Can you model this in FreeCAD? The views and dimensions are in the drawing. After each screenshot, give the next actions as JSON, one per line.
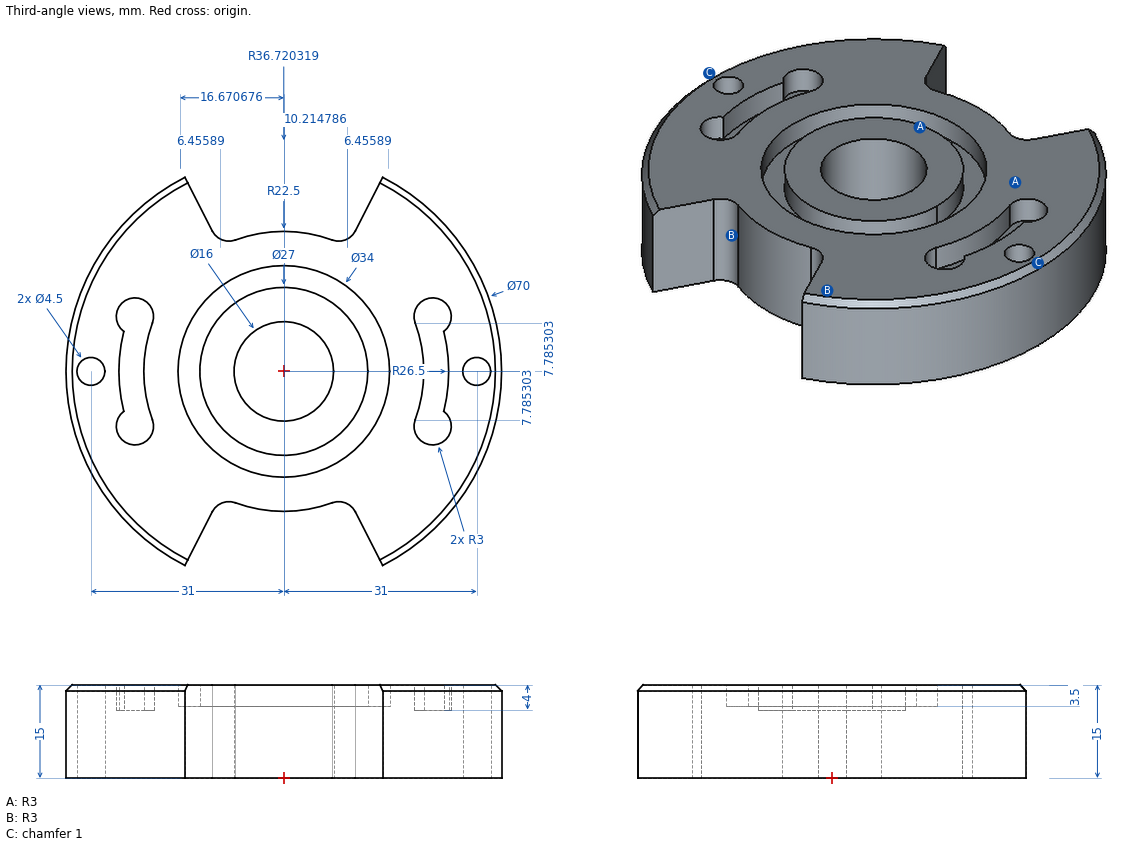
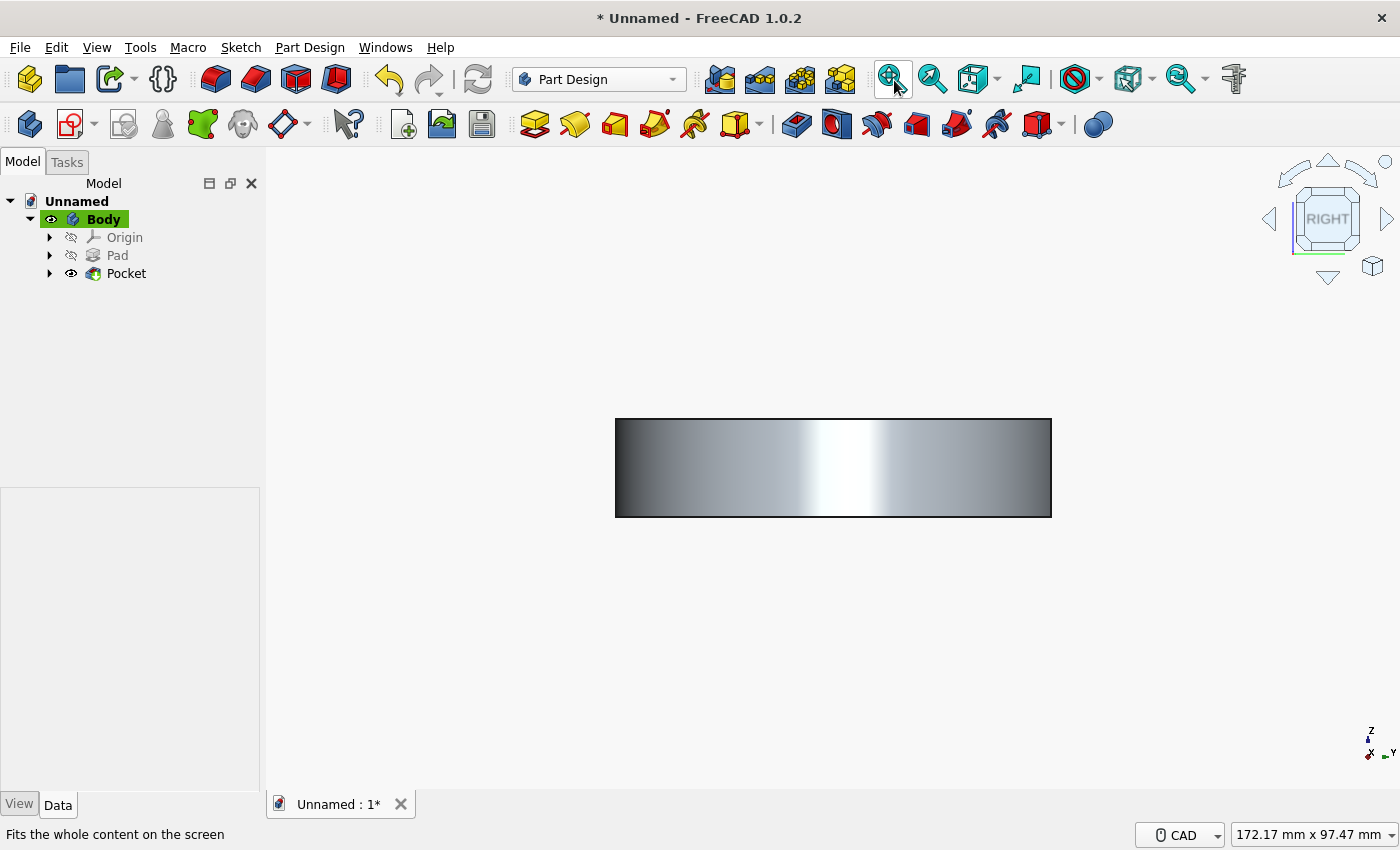
{"action": "key", "text": "5"}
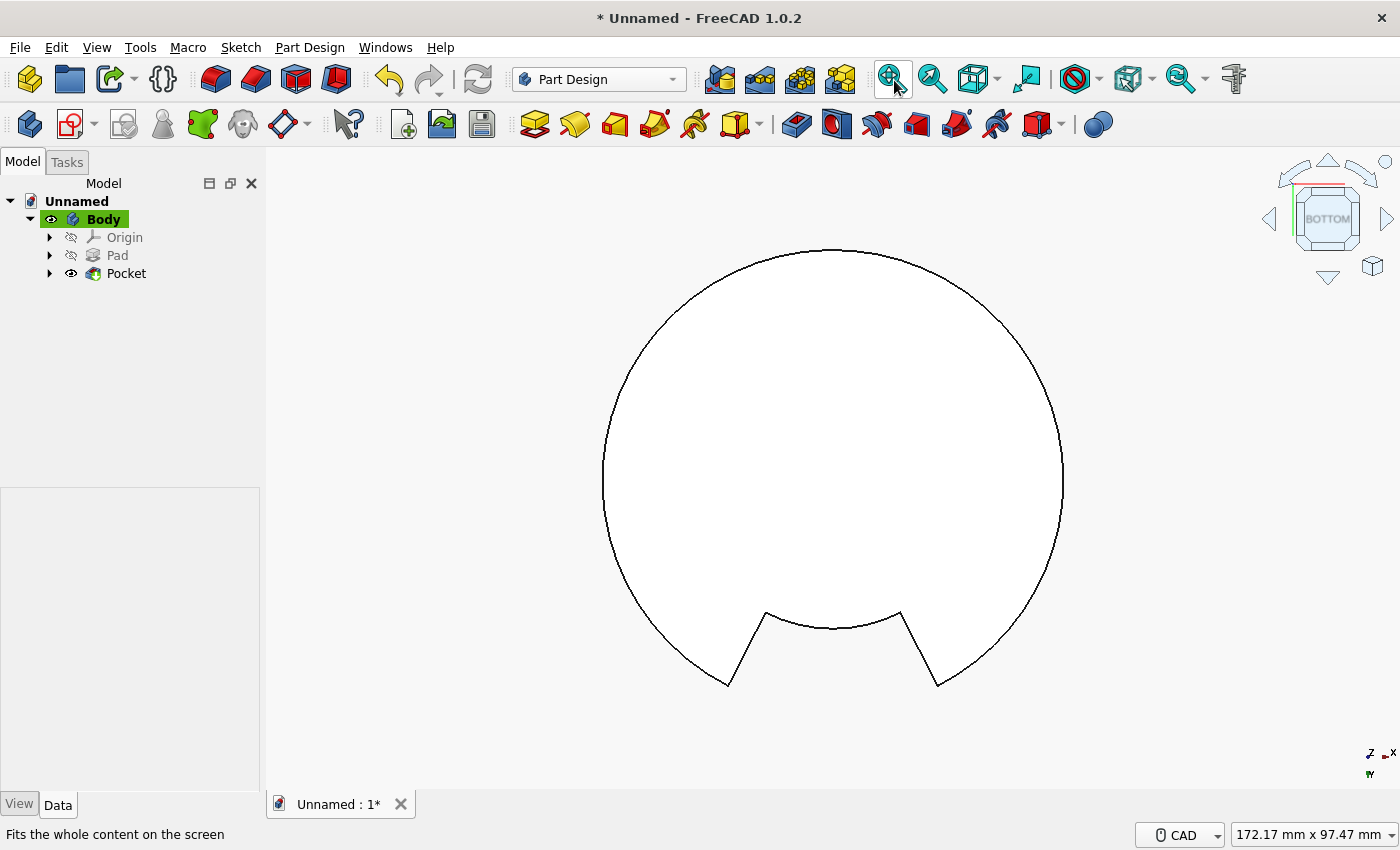
{"action": "key", "text": "4"}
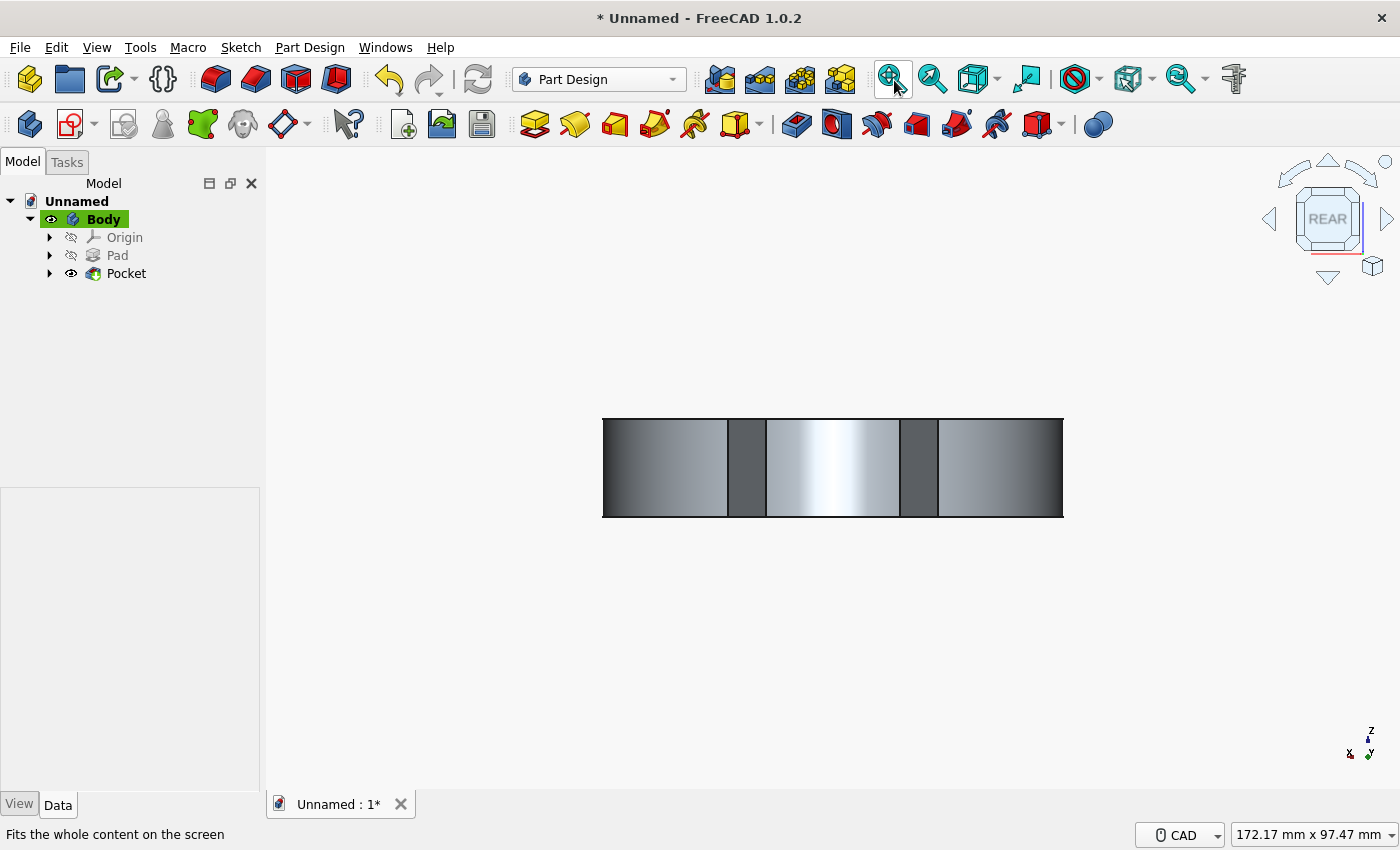
{"action": "key", "text": "v f"}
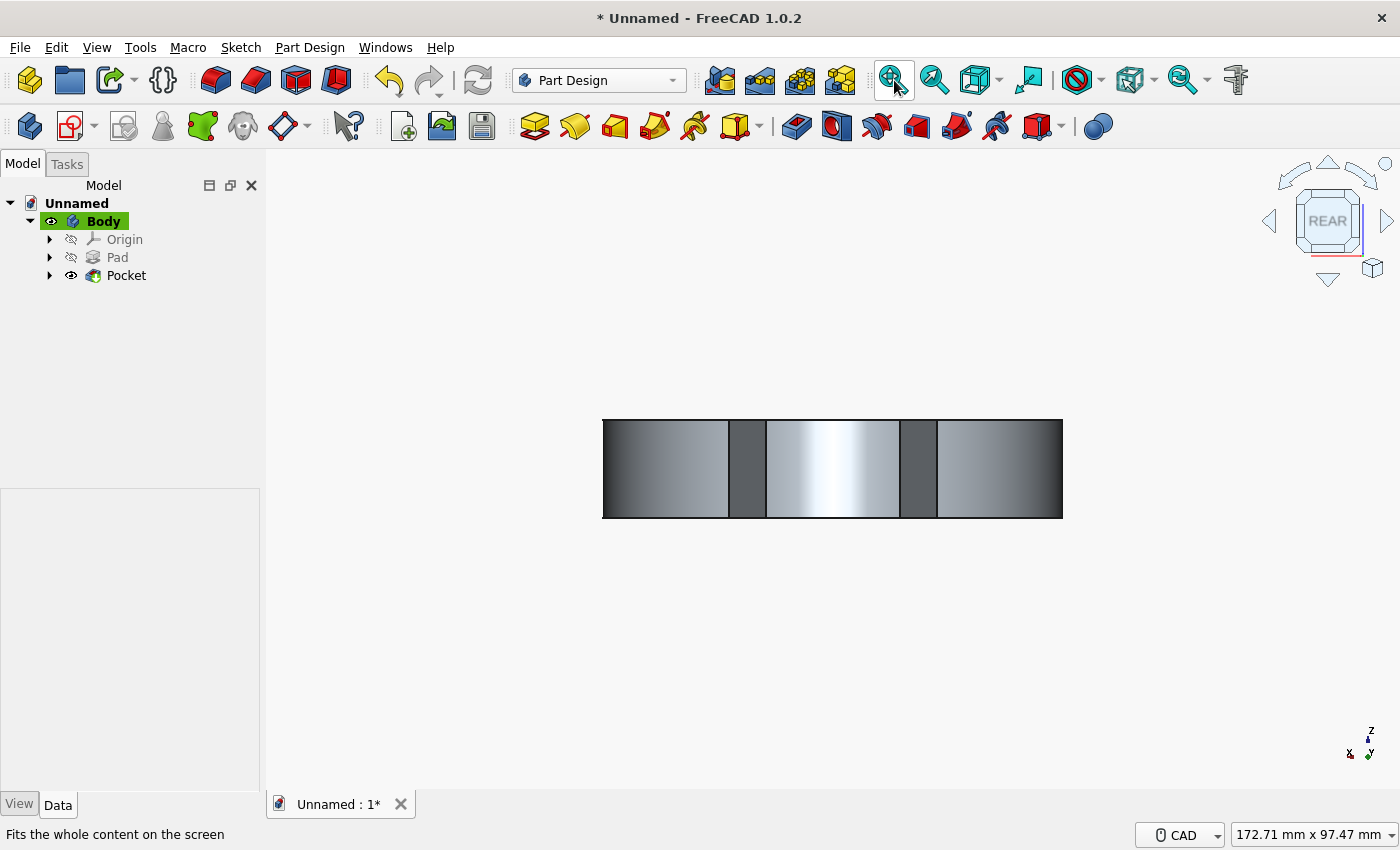
{"action": "key", "text": "6"}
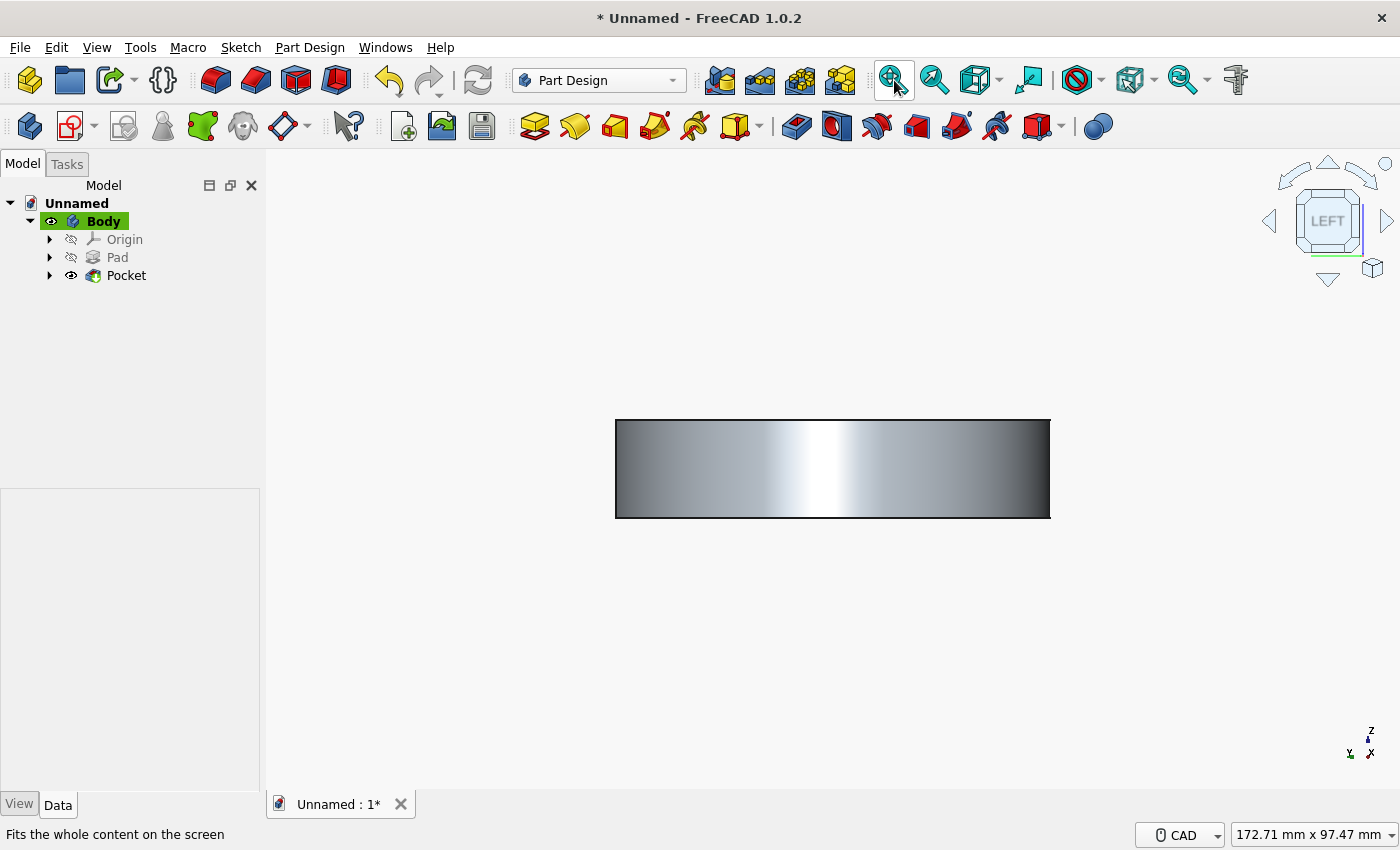
{"action": "left_click", "coordinate": [894, 80]}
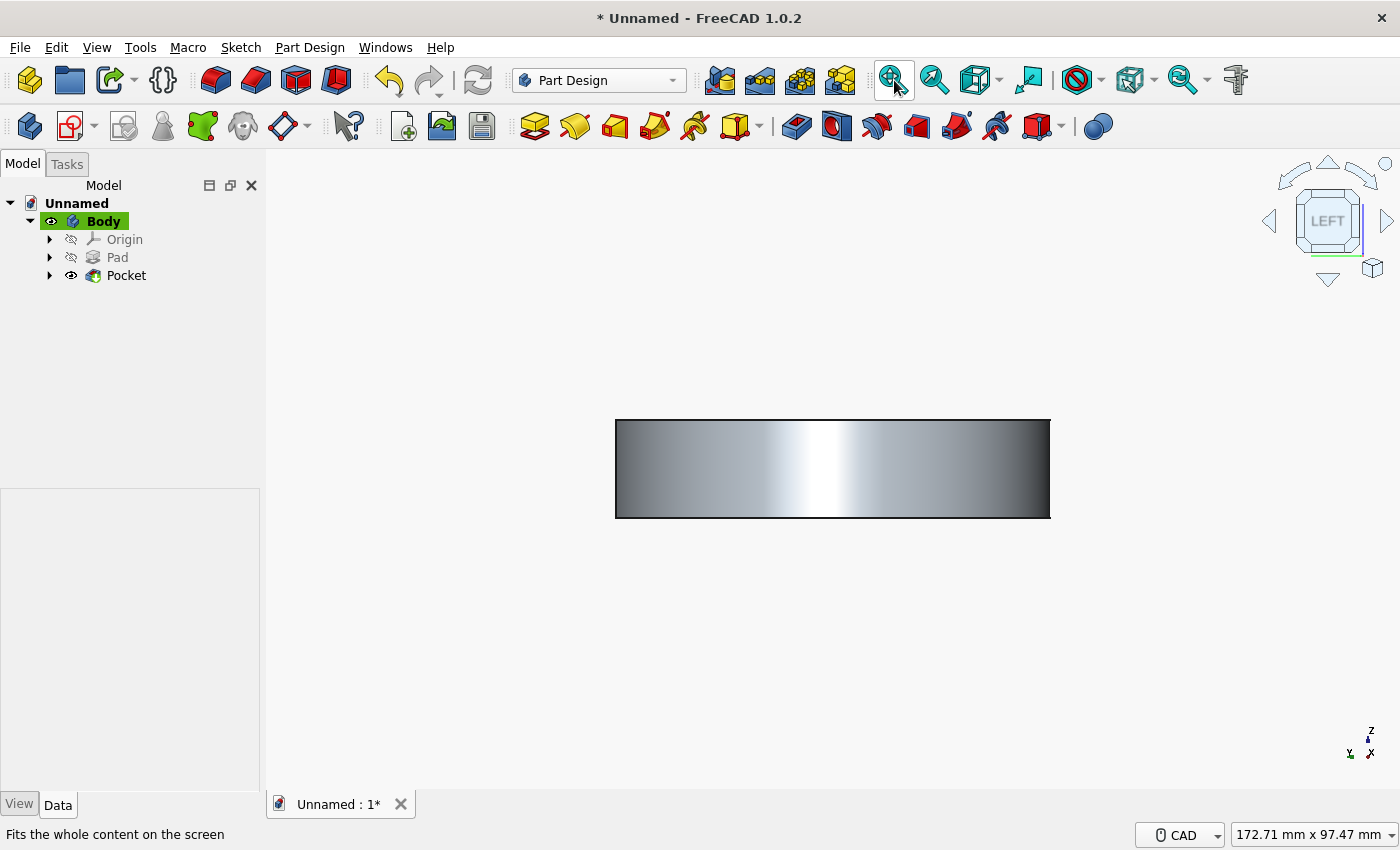
{"action": "key", "text": "v 3"}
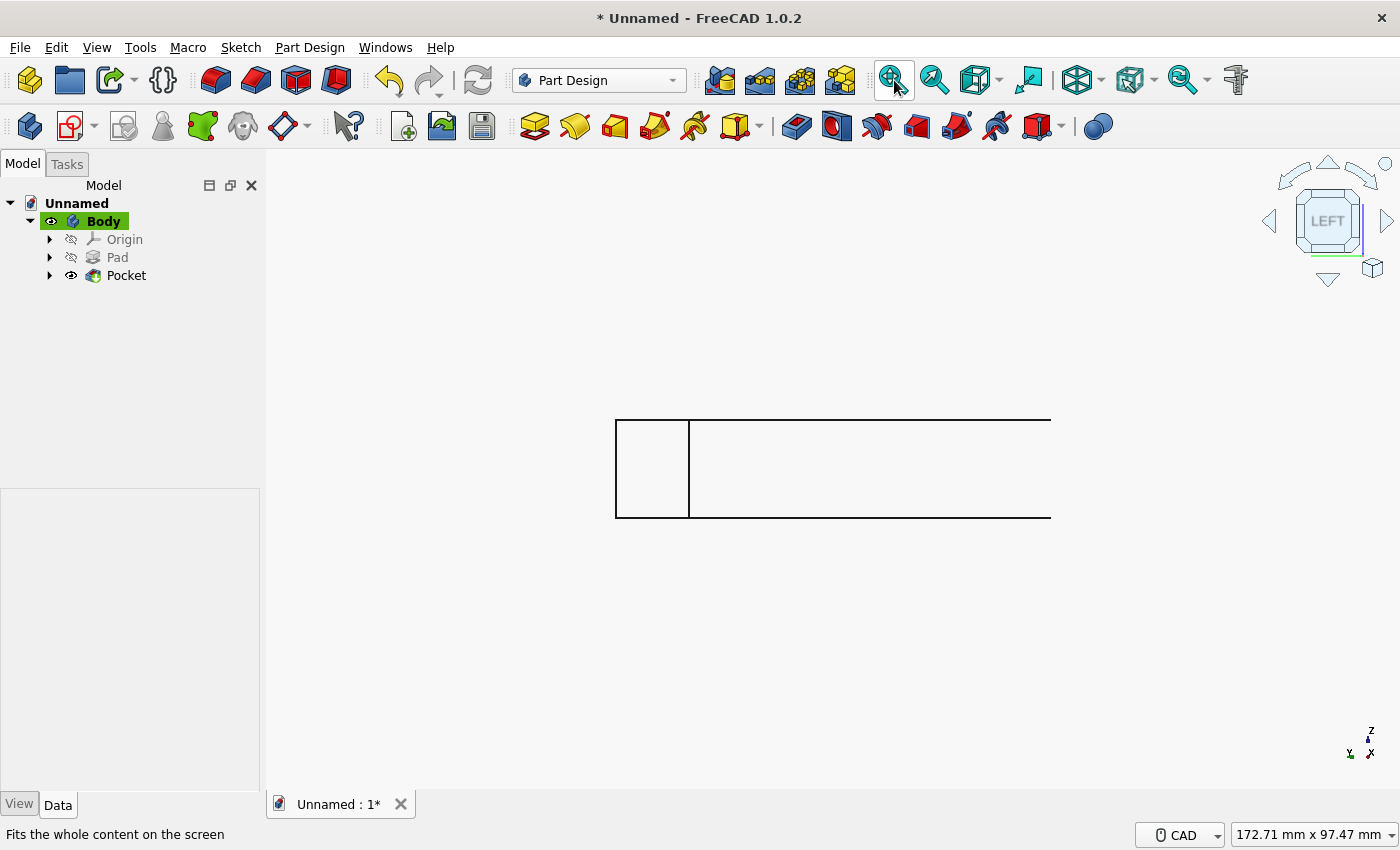
{"action": "key", "text": "0"}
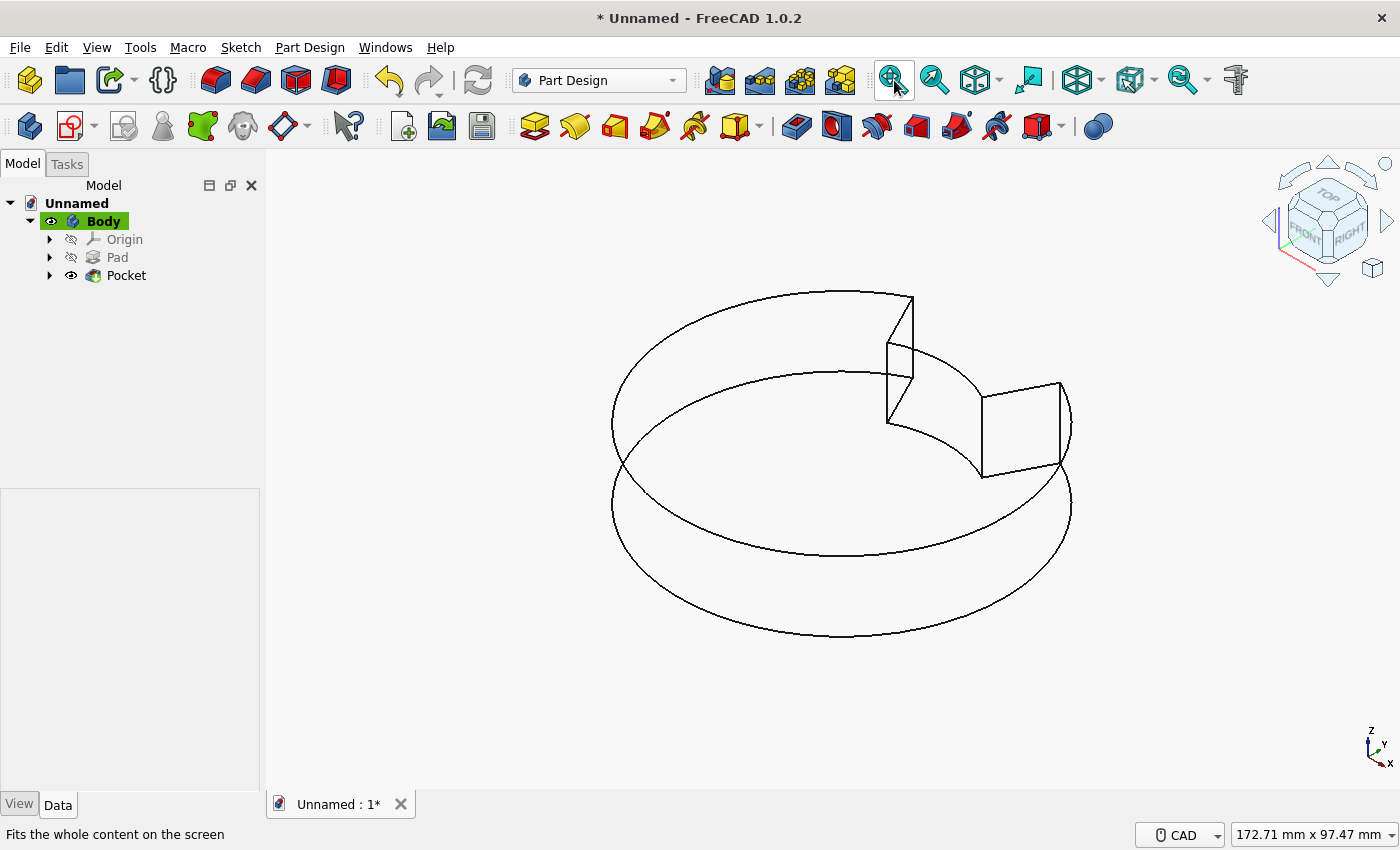
{"action": "left_click", "coordinate": [887, 382]}